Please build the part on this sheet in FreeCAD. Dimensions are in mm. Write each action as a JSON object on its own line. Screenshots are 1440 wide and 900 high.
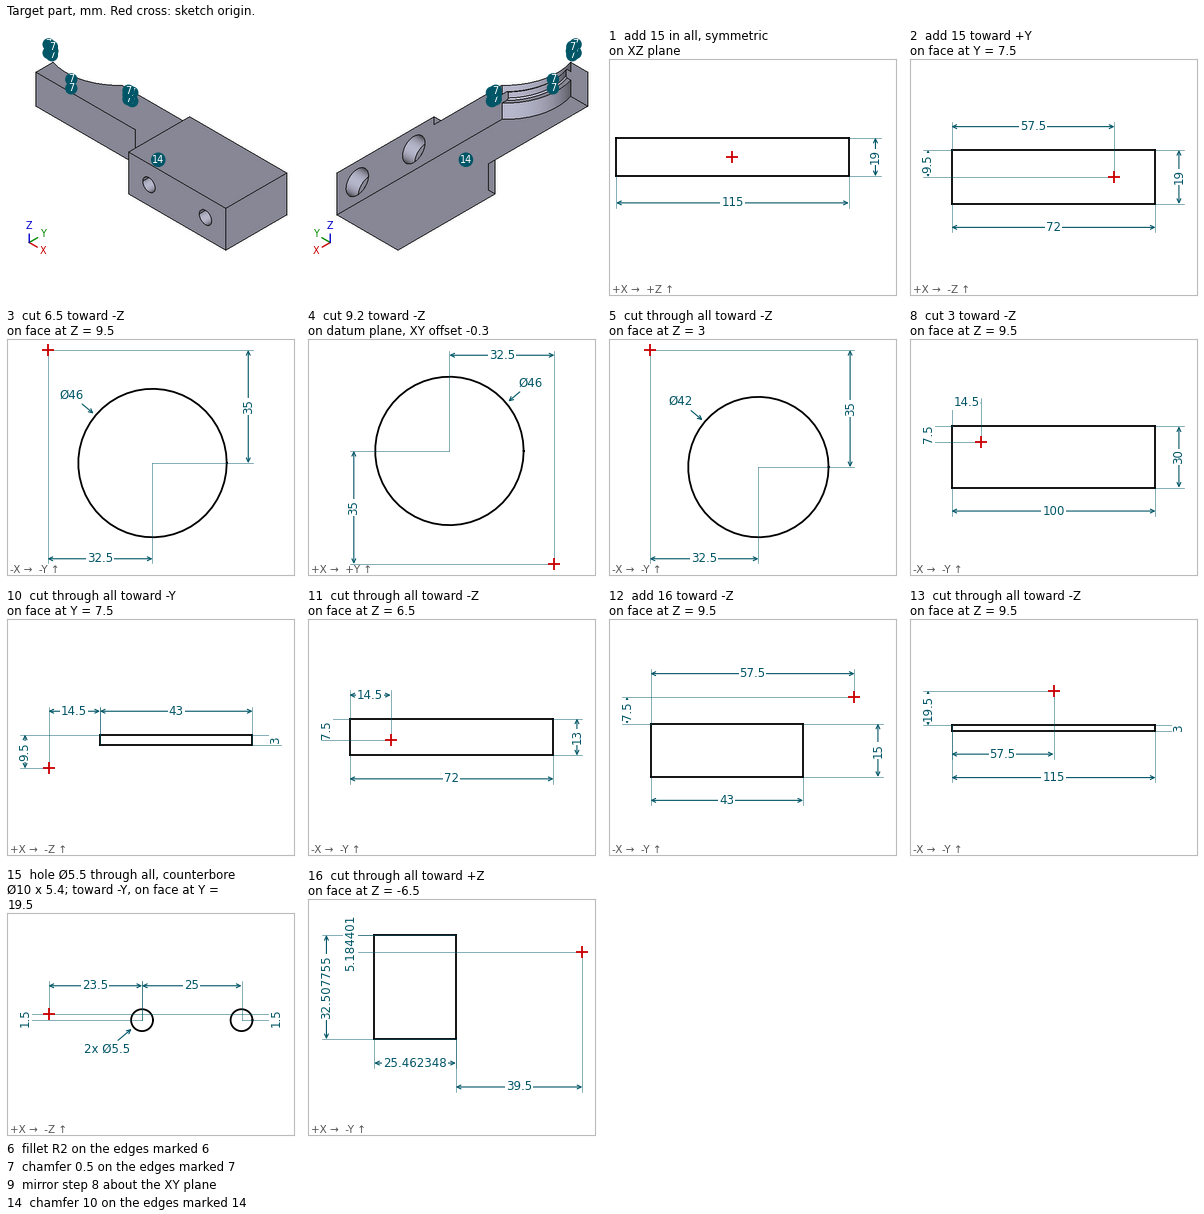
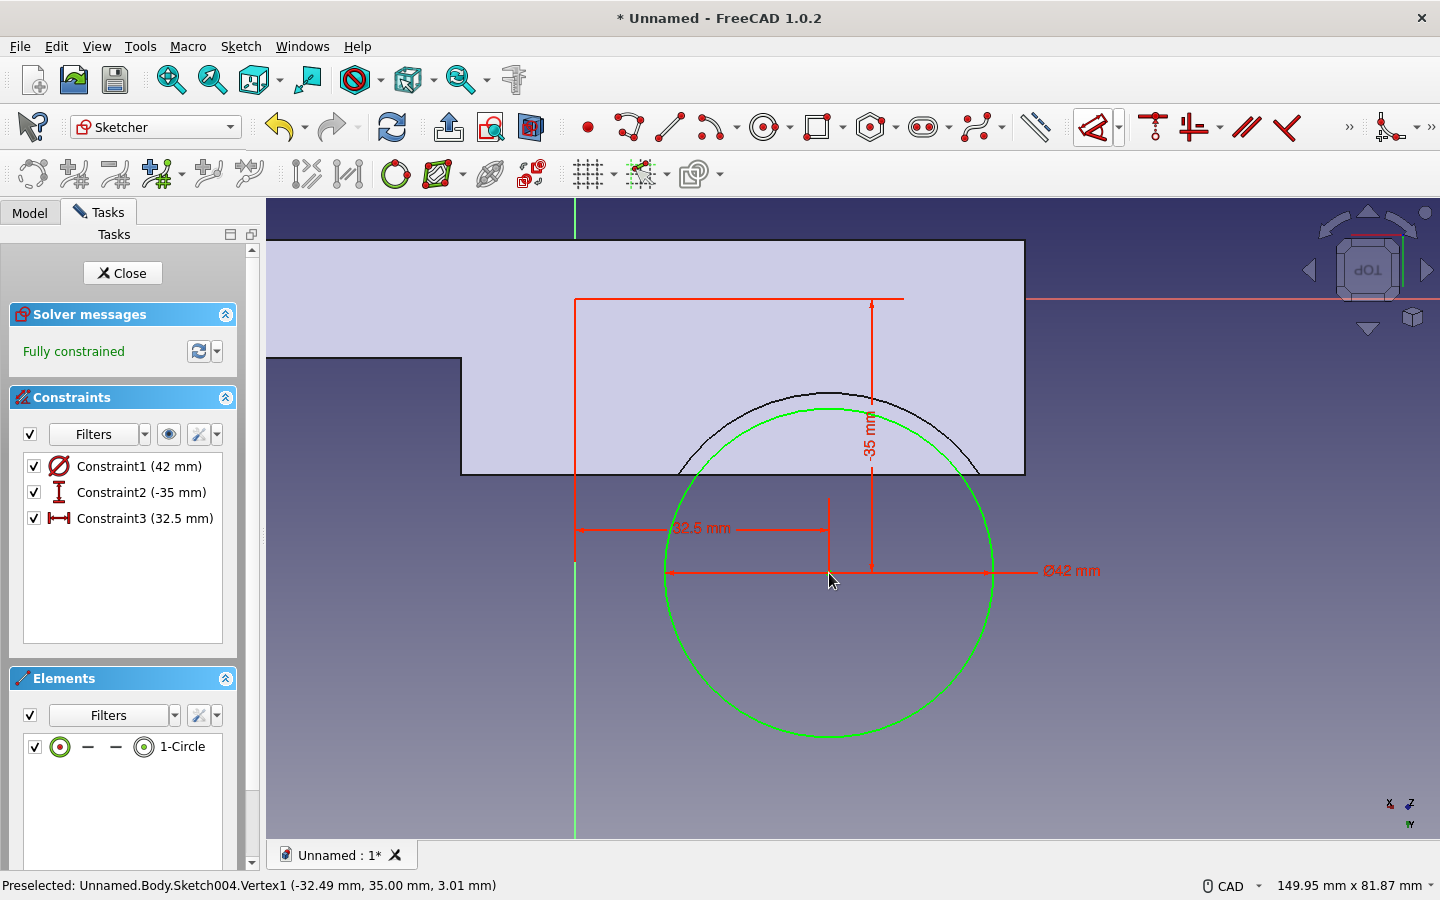
{"action": "left_click", "coordinate": [123, 273]}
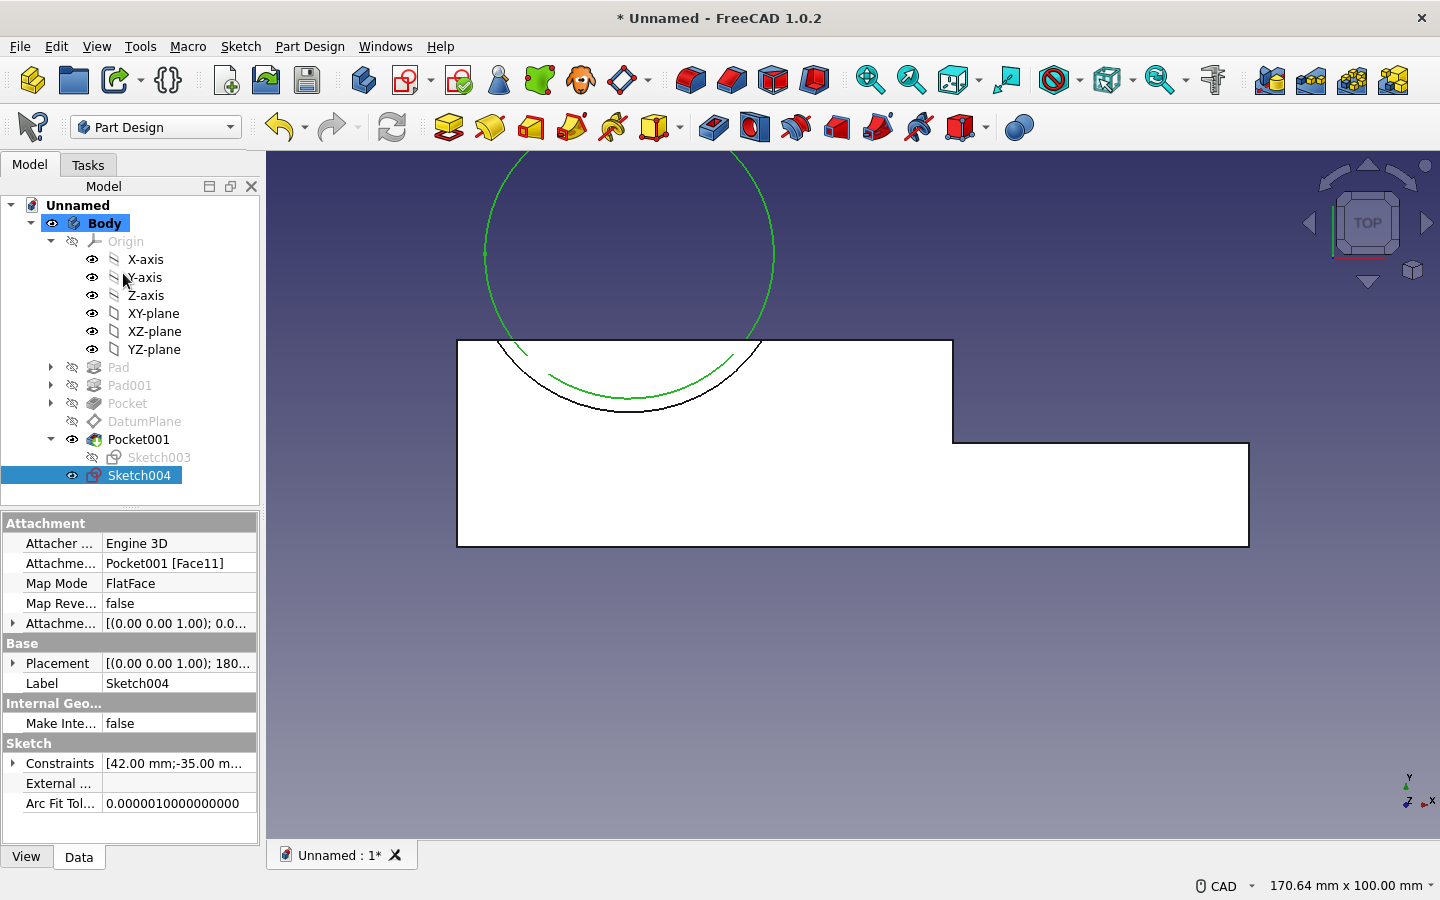
{"action": "left_click", "coordinate": [714, 128]}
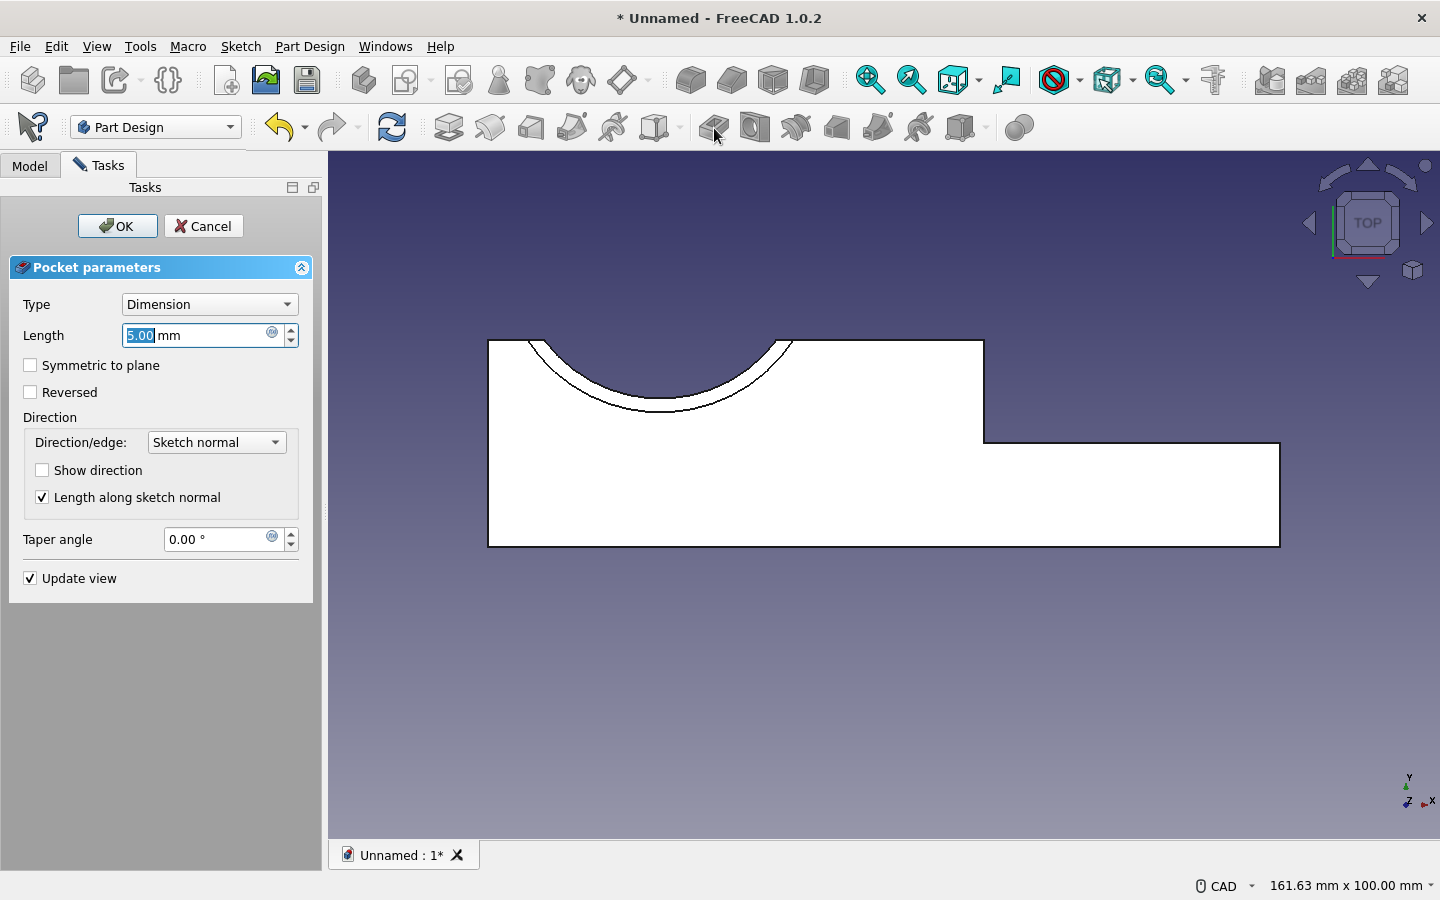
{"action": "left_click", "coordinate": [210, 304]}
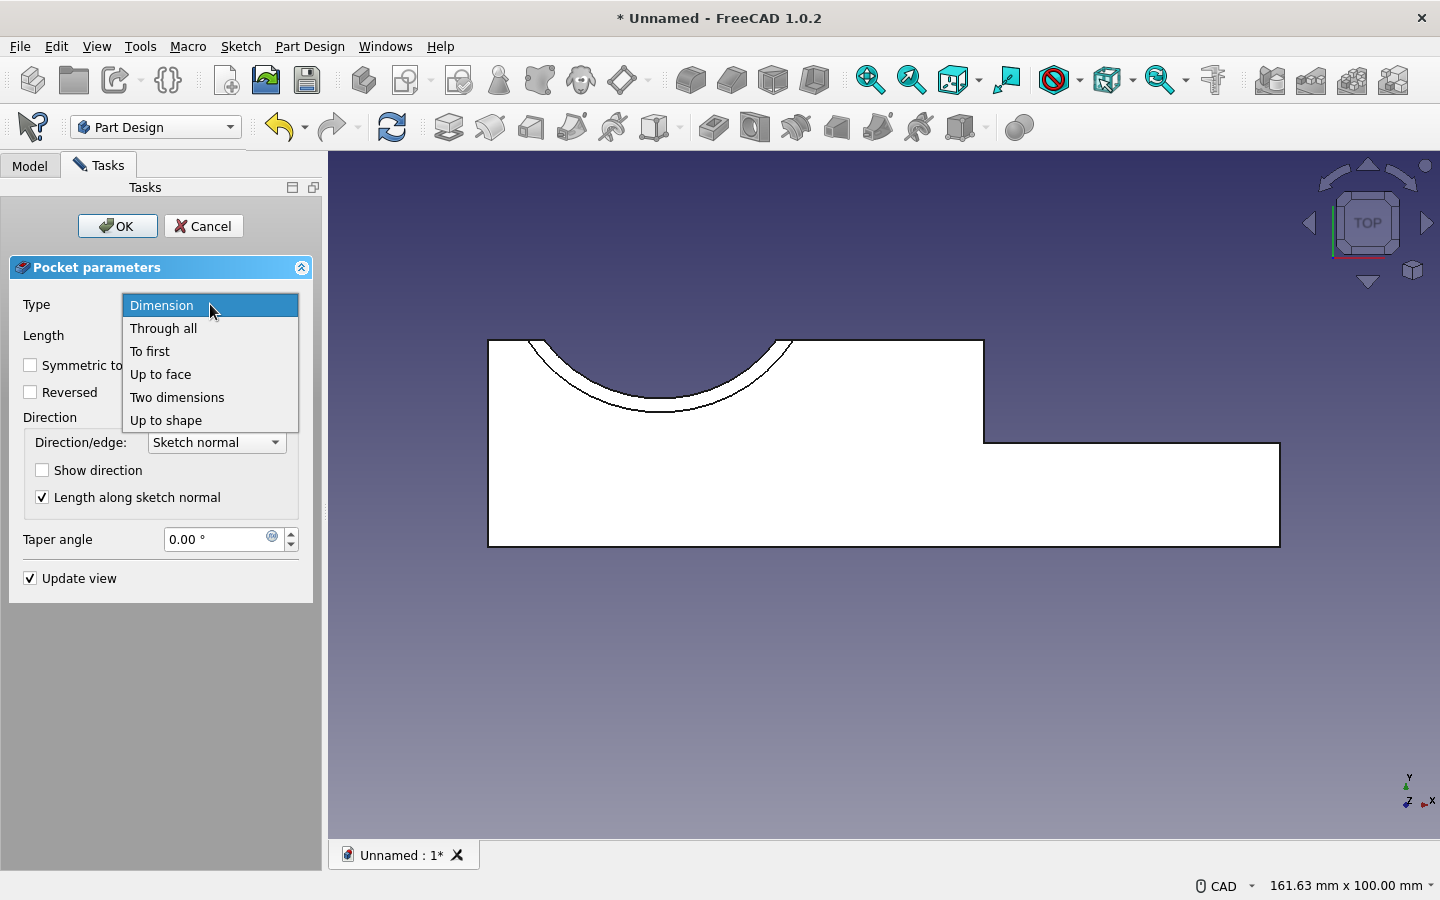
{"action": "left_click", "coordinate": [208, 328]}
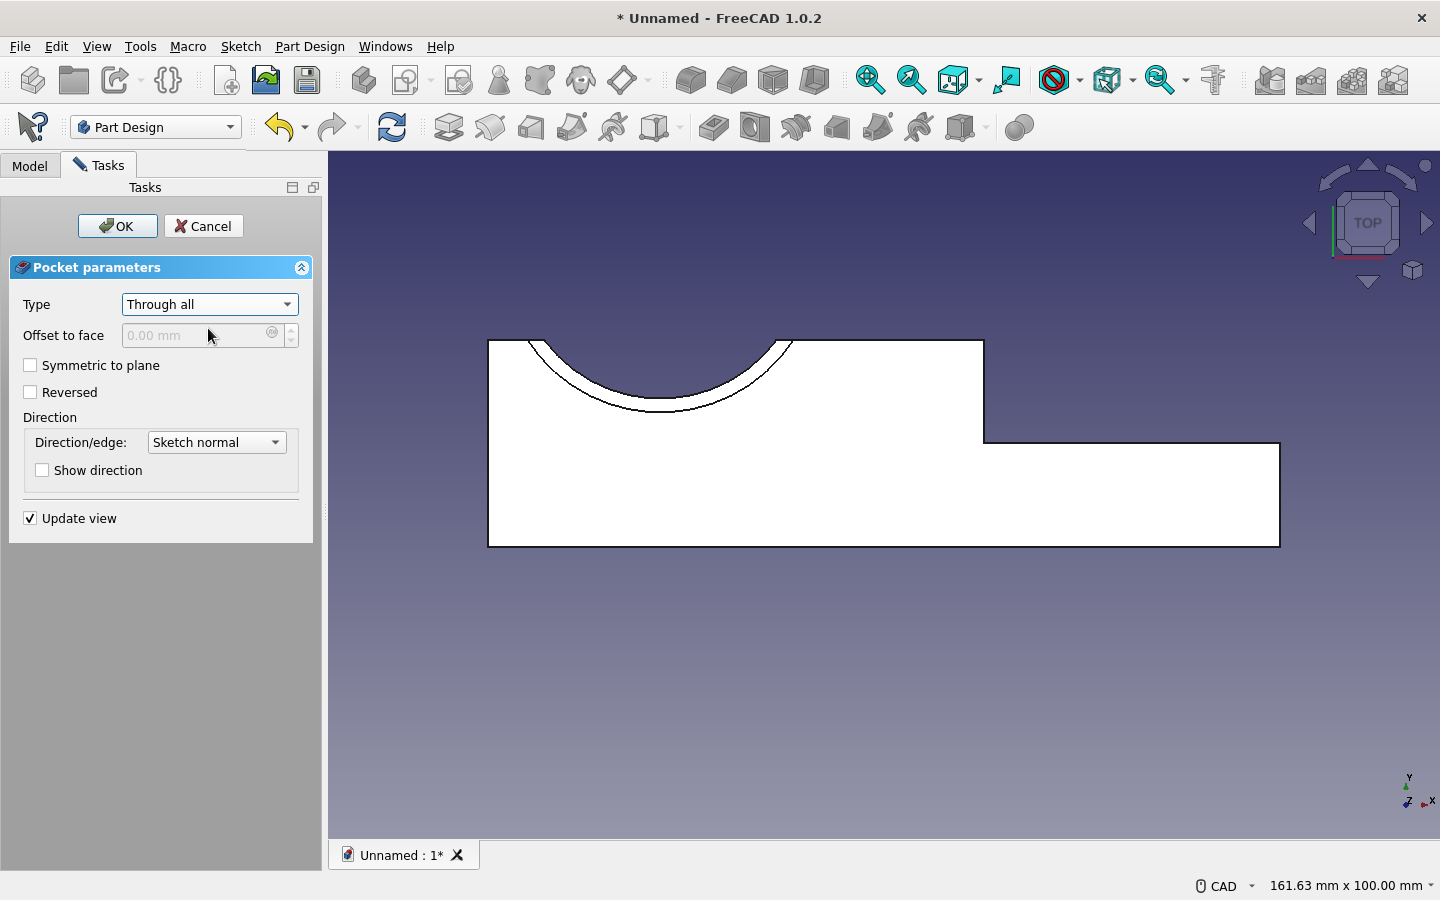
{"action": "left_click", "coordinate": [118, 226]}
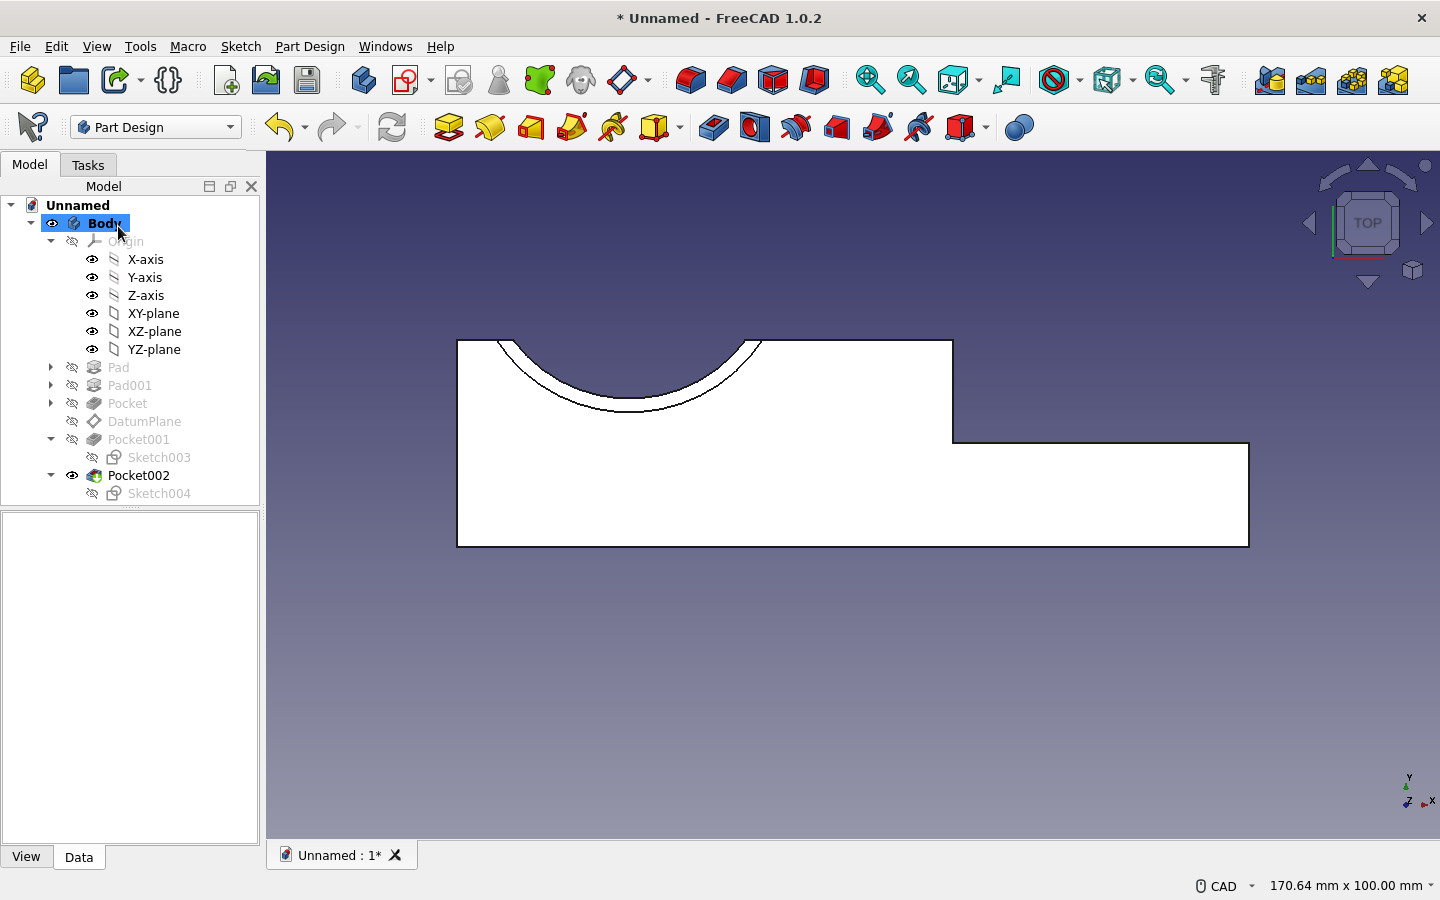
{"action": "key", "text": "0"}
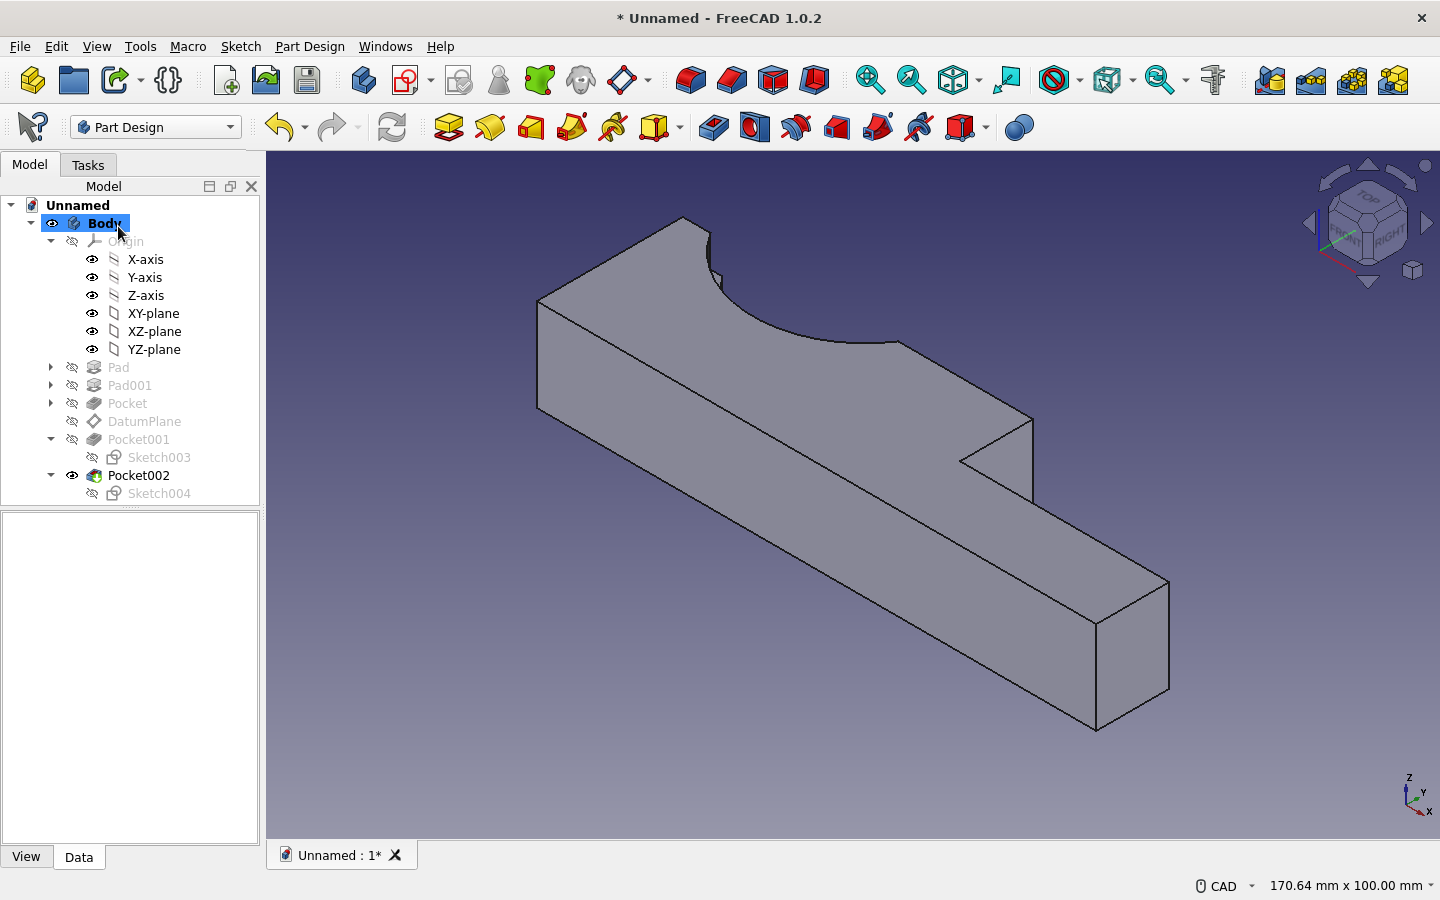
{"action": "key", "text": "2"}